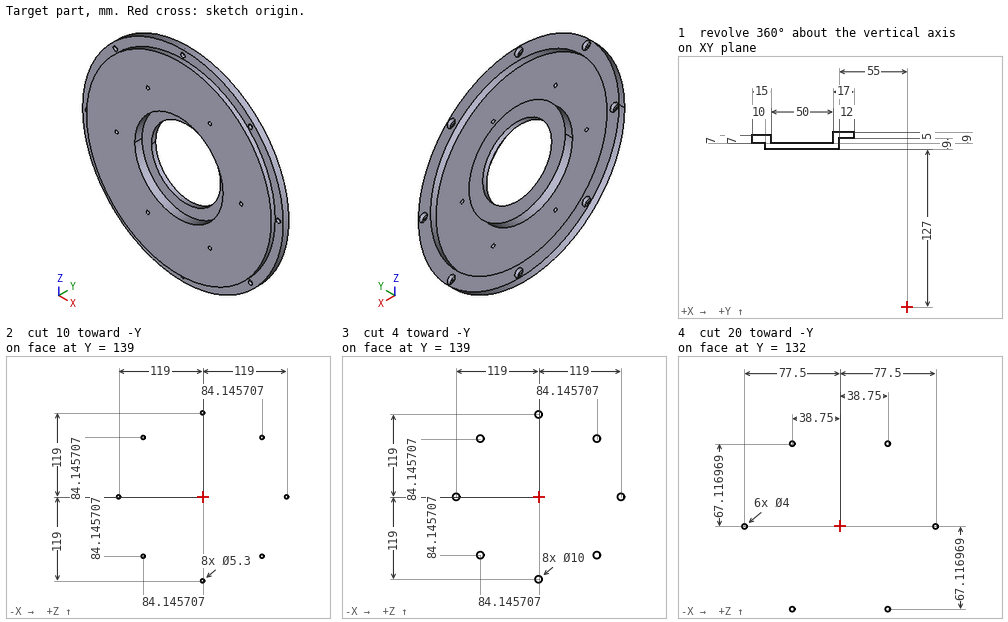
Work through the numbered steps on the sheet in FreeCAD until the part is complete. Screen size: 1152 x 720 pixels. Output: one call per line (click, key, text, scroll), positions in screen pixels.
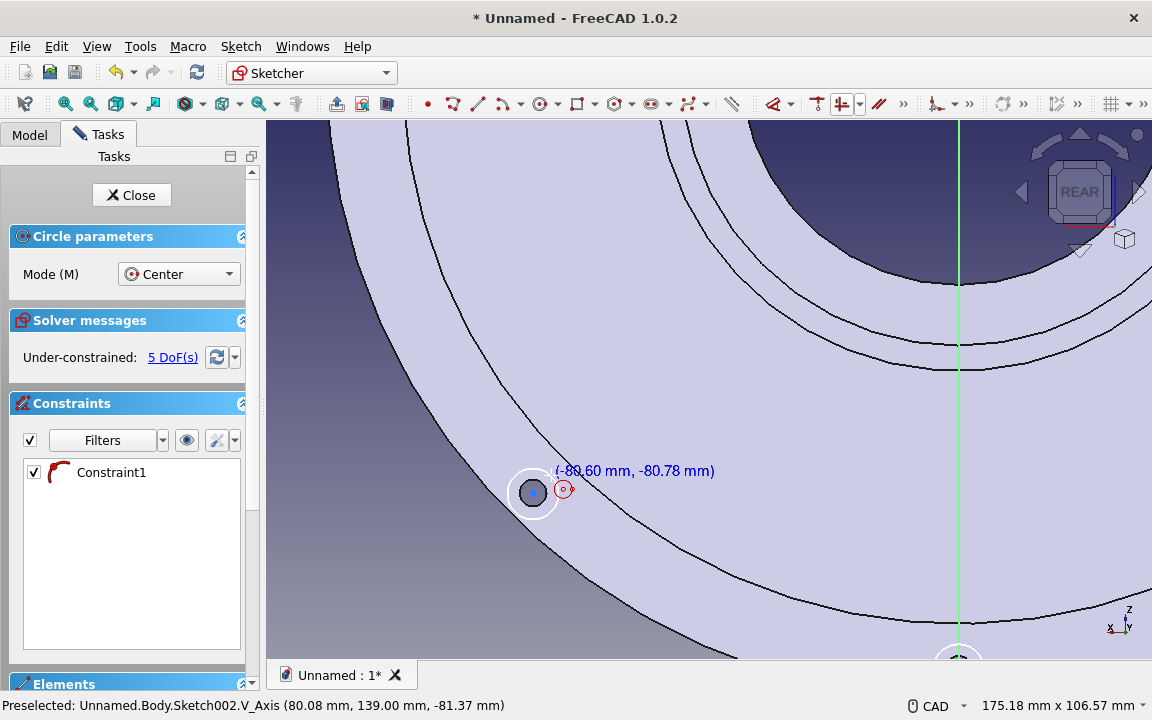
scroll(536, 495, down, 7)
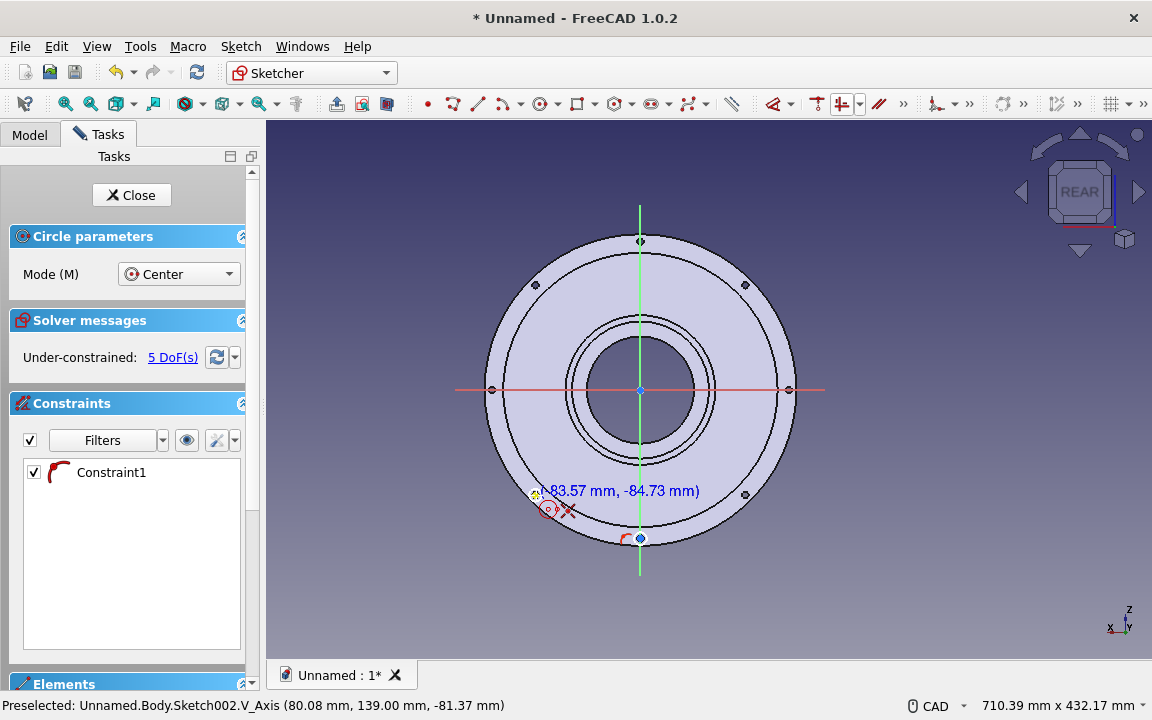
scroll(492, 390, up, 7)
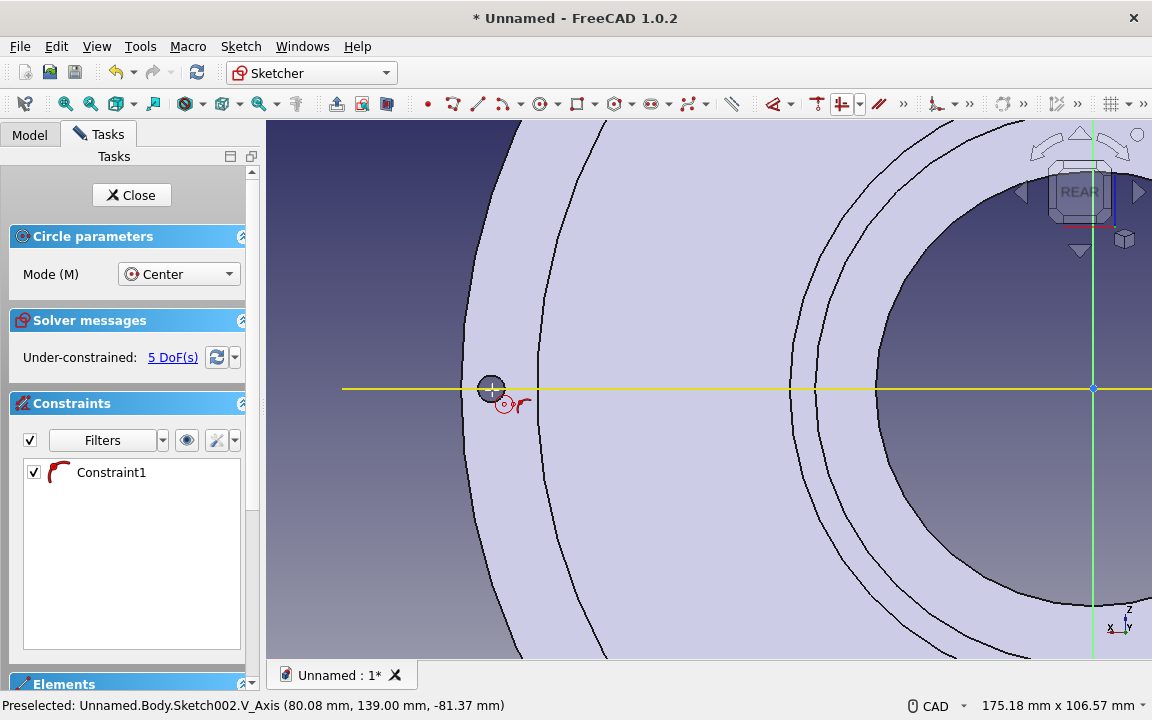
click(491, 389)
click(509, 371)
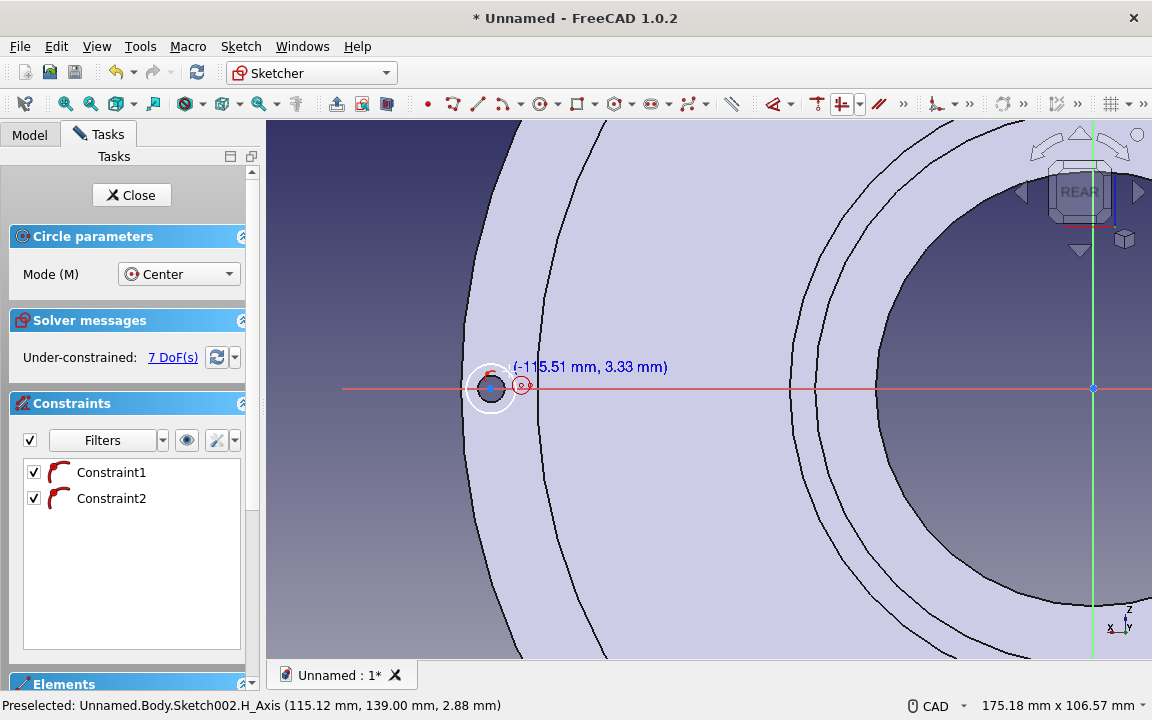
scroll(492, 390, down, 7)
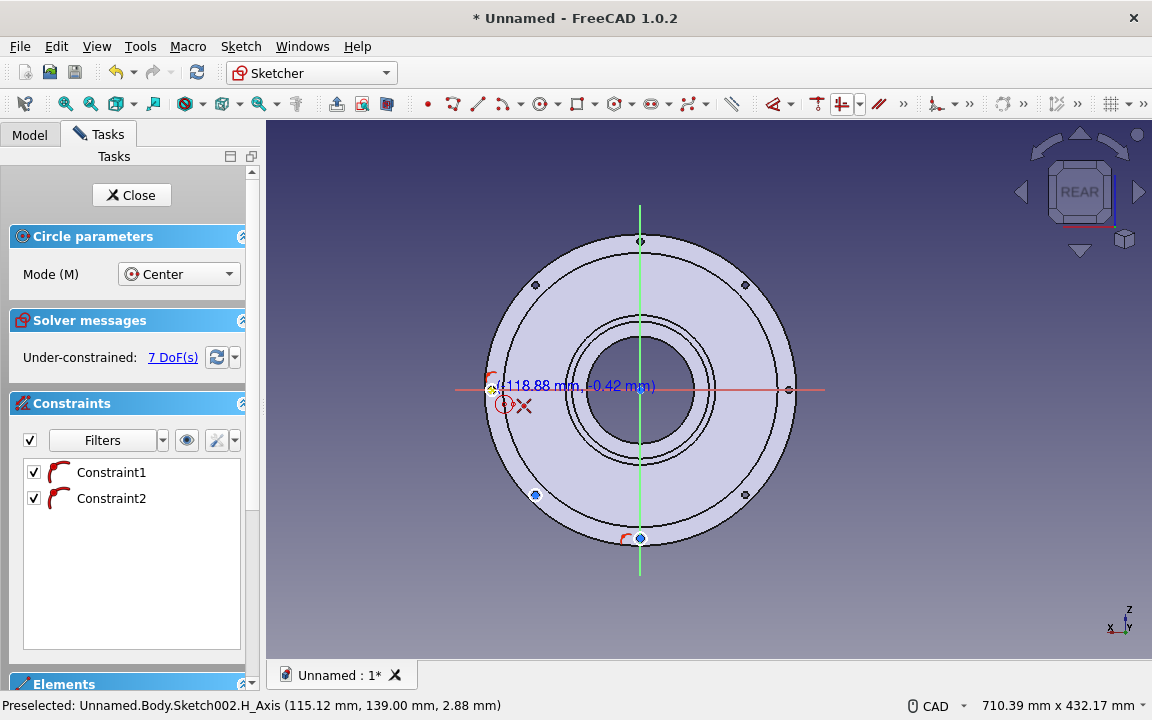
scroll(536, 285, up, 7)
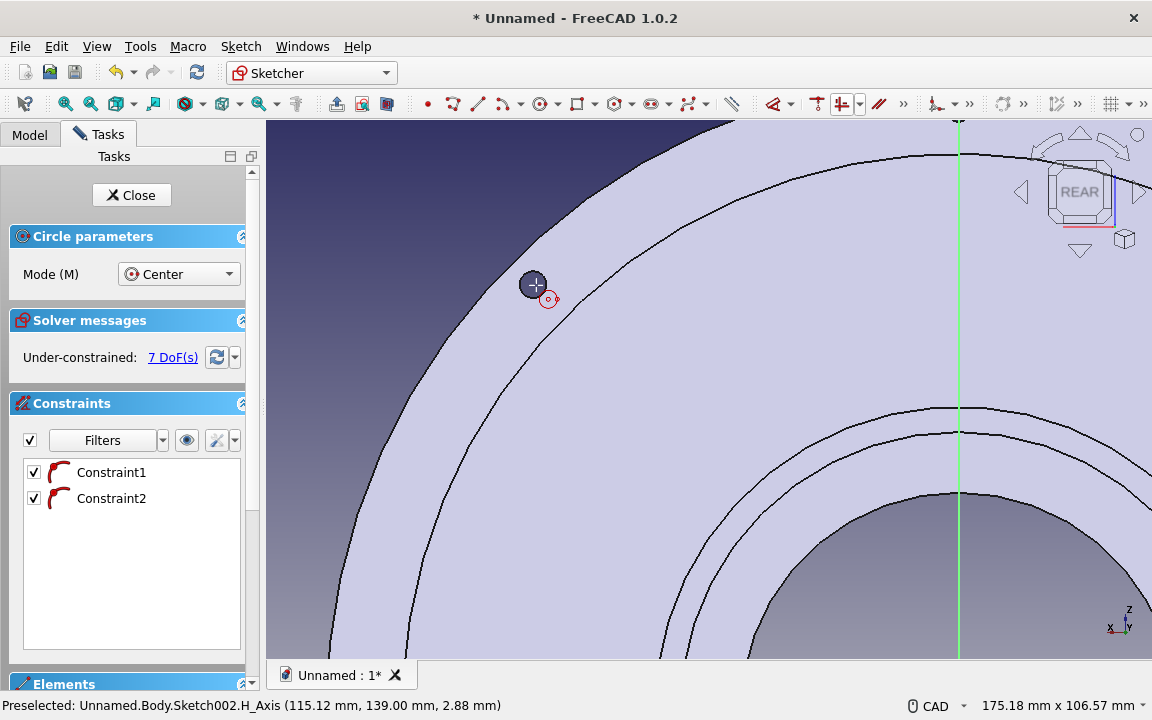
click(533, 285)
click(551, 267)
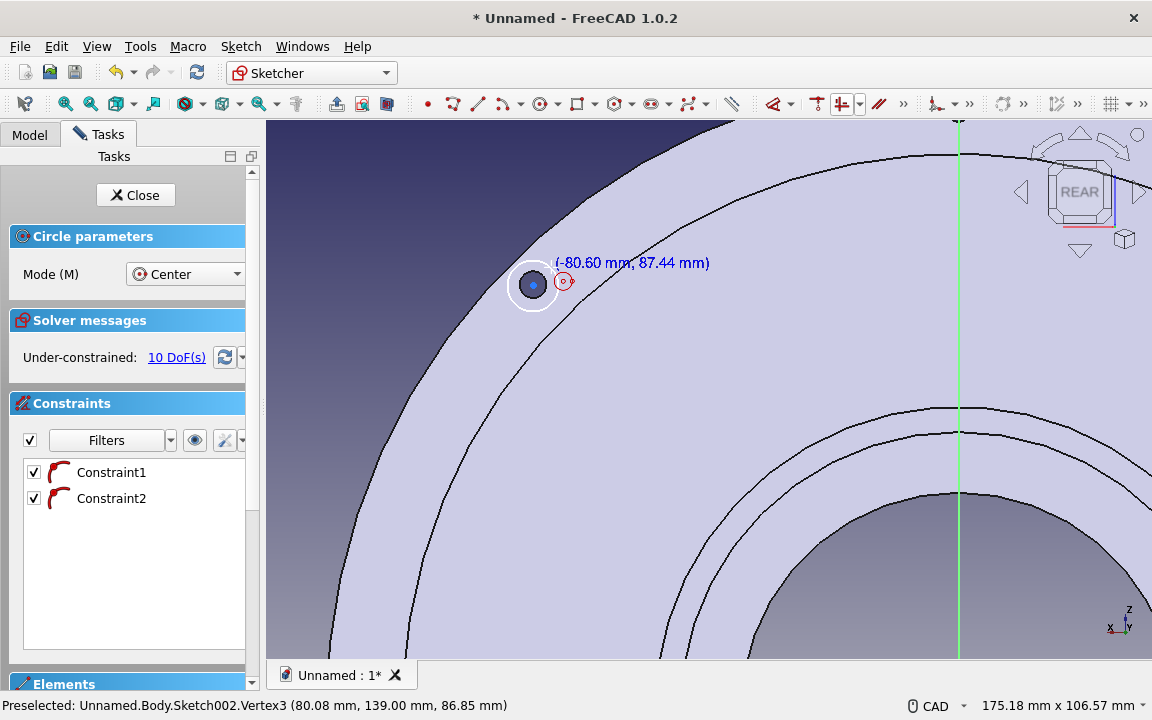
scroll(536, 285, down, 7)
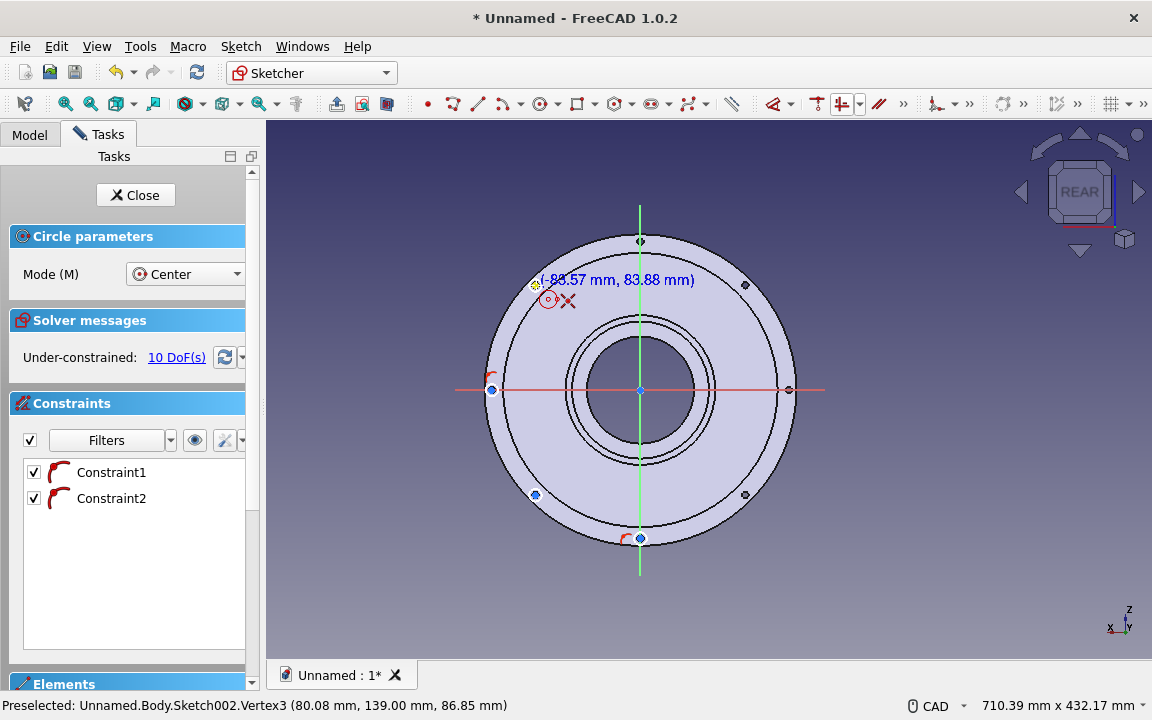
scroll(640, 242, up, 7)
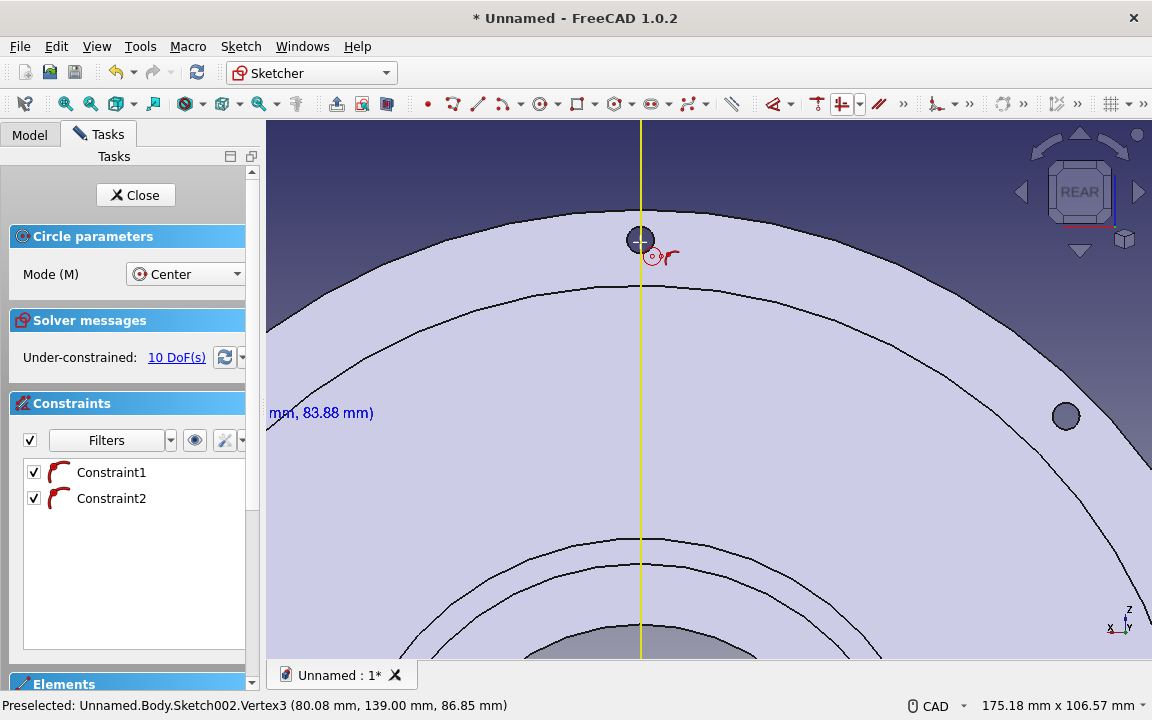
click(641, 240)
click(658, 222)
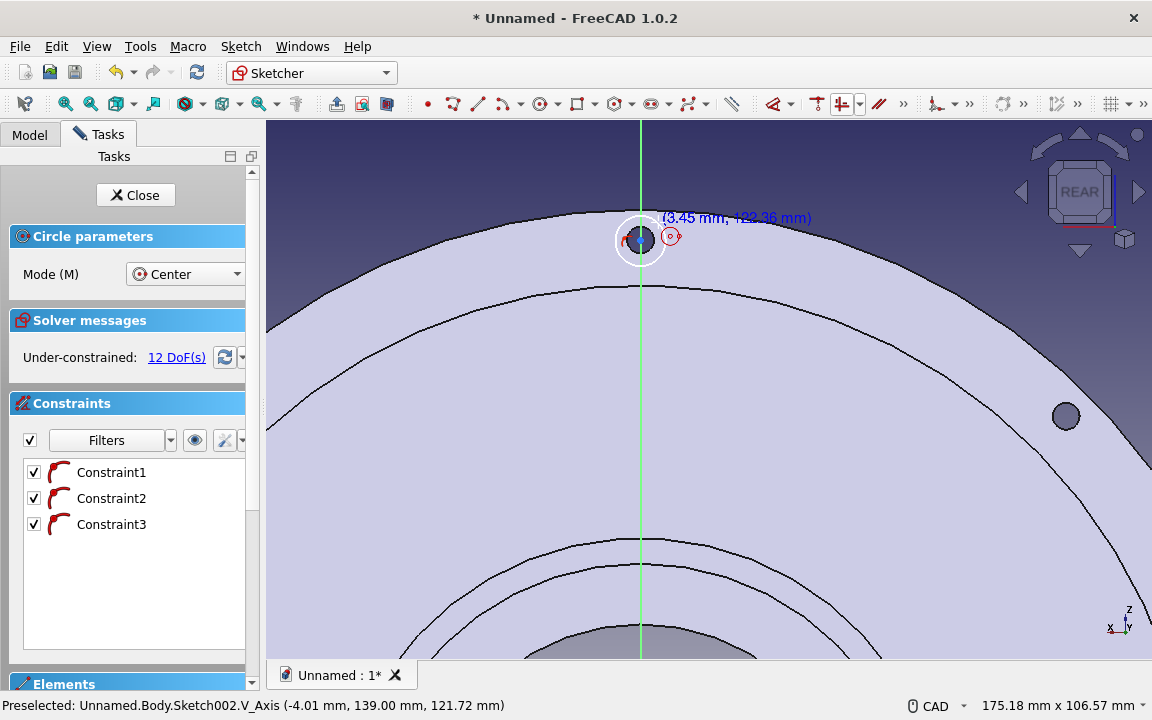
scroll(640, 241, down, 7)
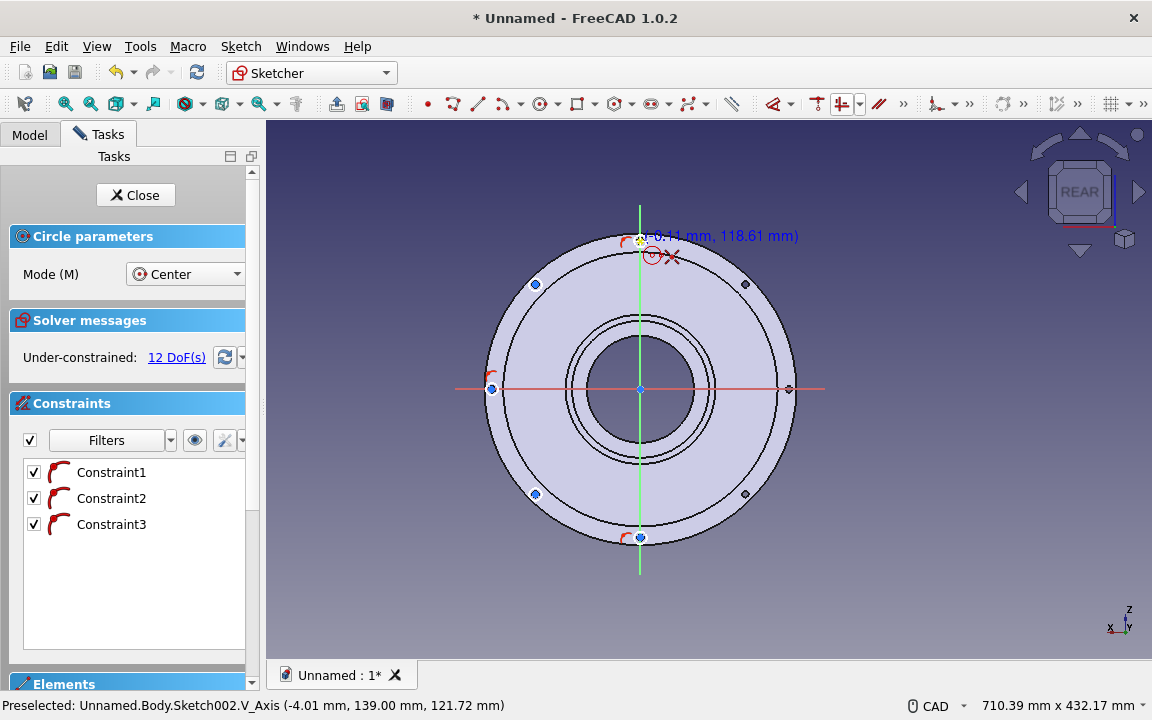
scroll(745, 284, up, 7)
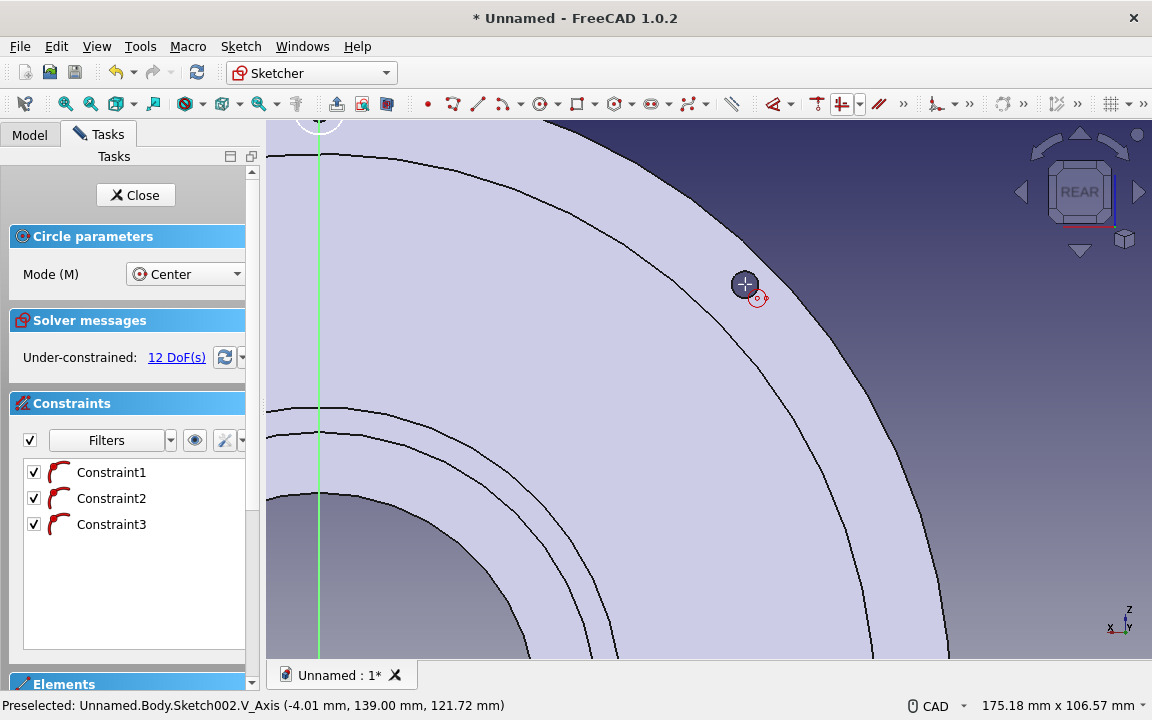
click(745, 285)
click(763, 267)